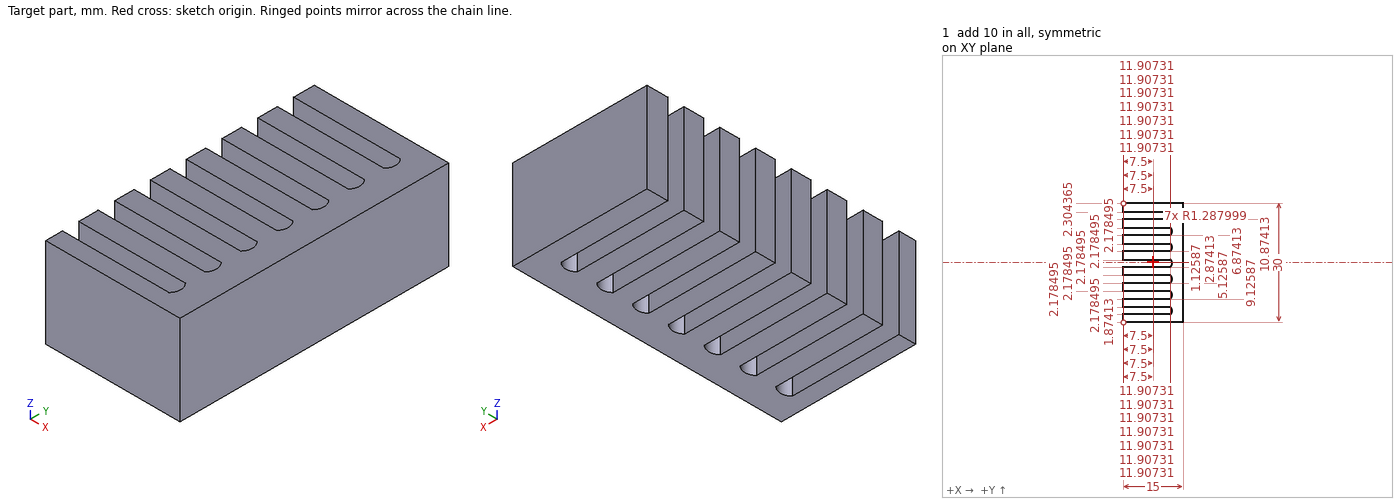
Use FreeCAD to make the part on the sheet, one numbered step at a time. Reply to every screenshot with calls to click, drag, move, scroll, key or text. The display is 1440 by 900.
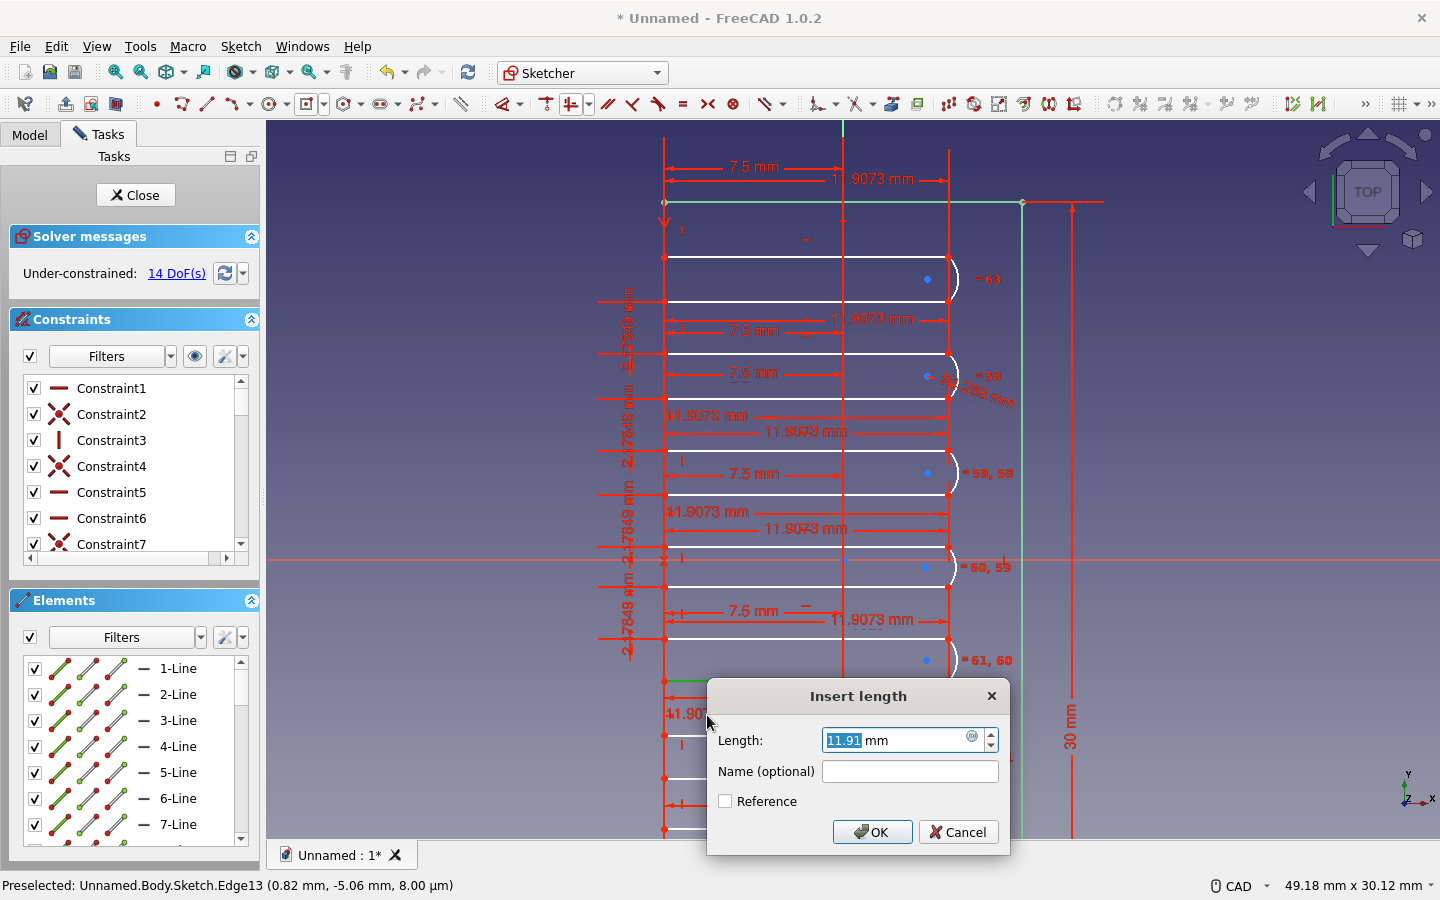
text(11.90731)
key(Return)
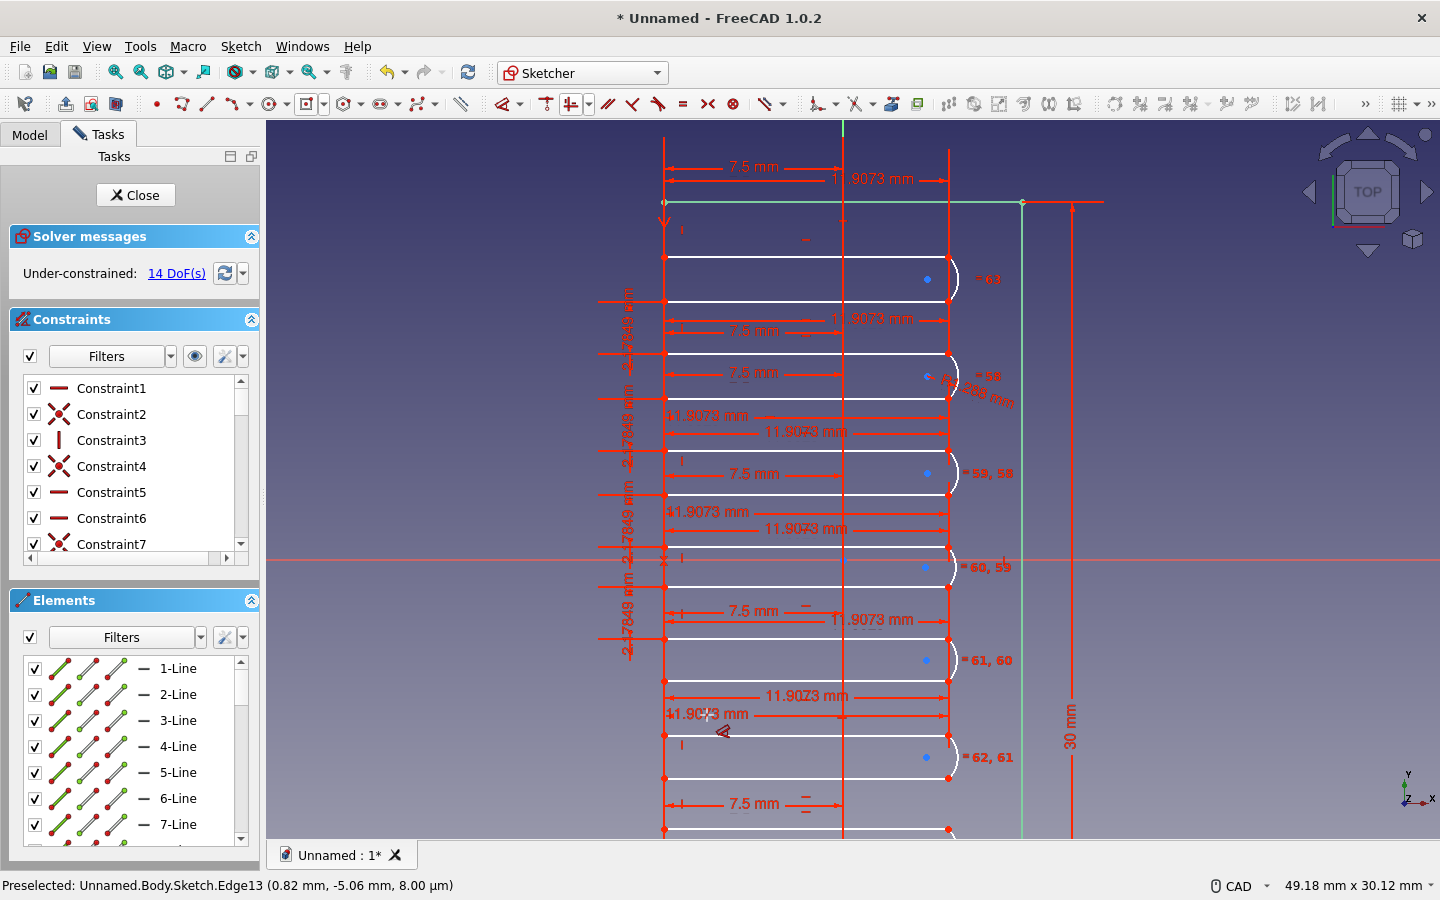
click(664, 698)
click(630, 709)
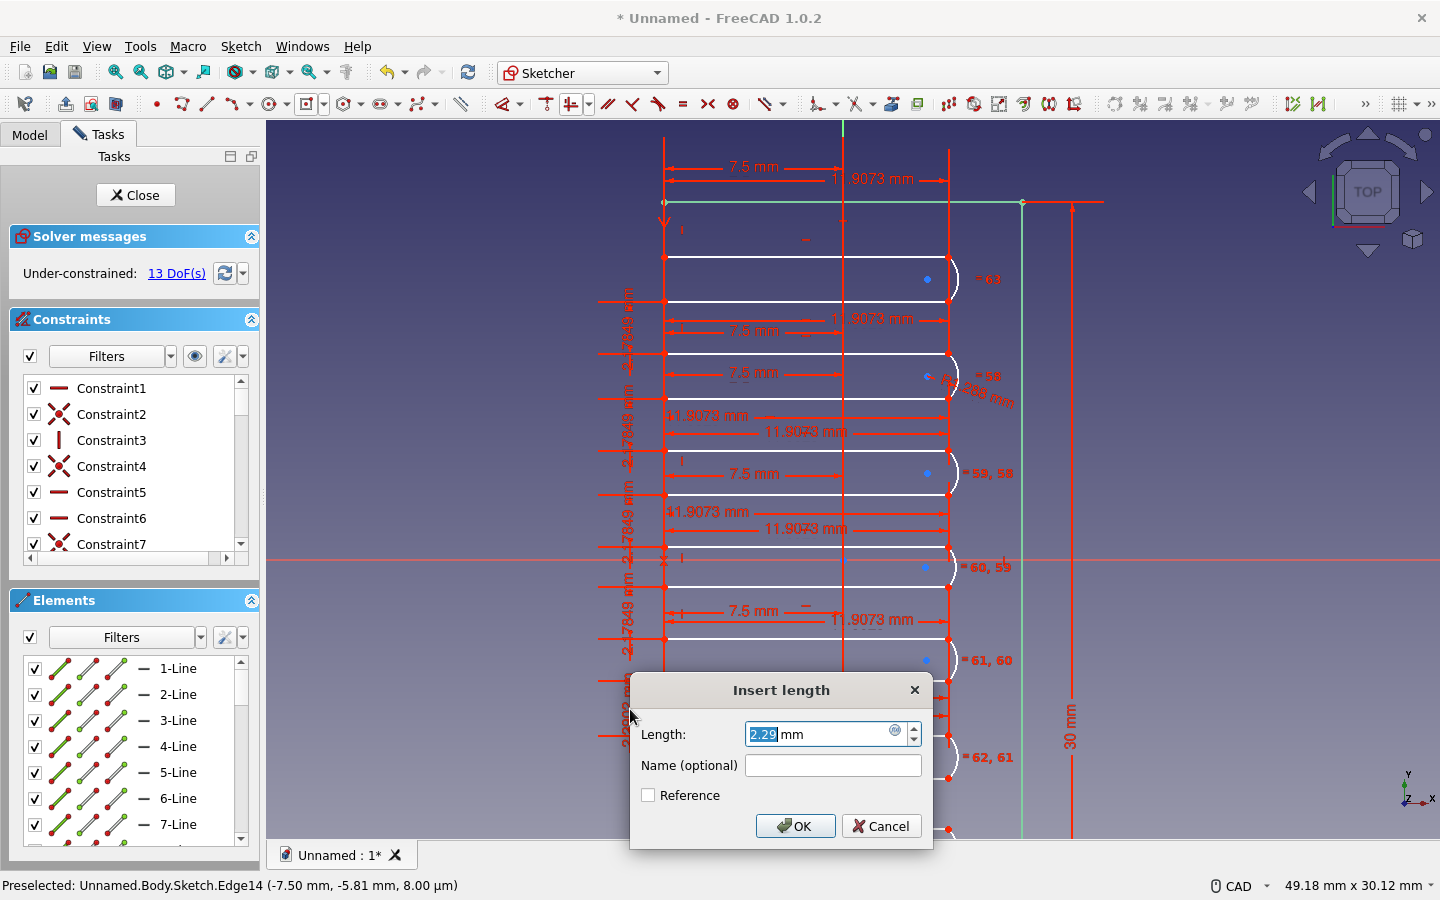
text(2.178495)
key(Return)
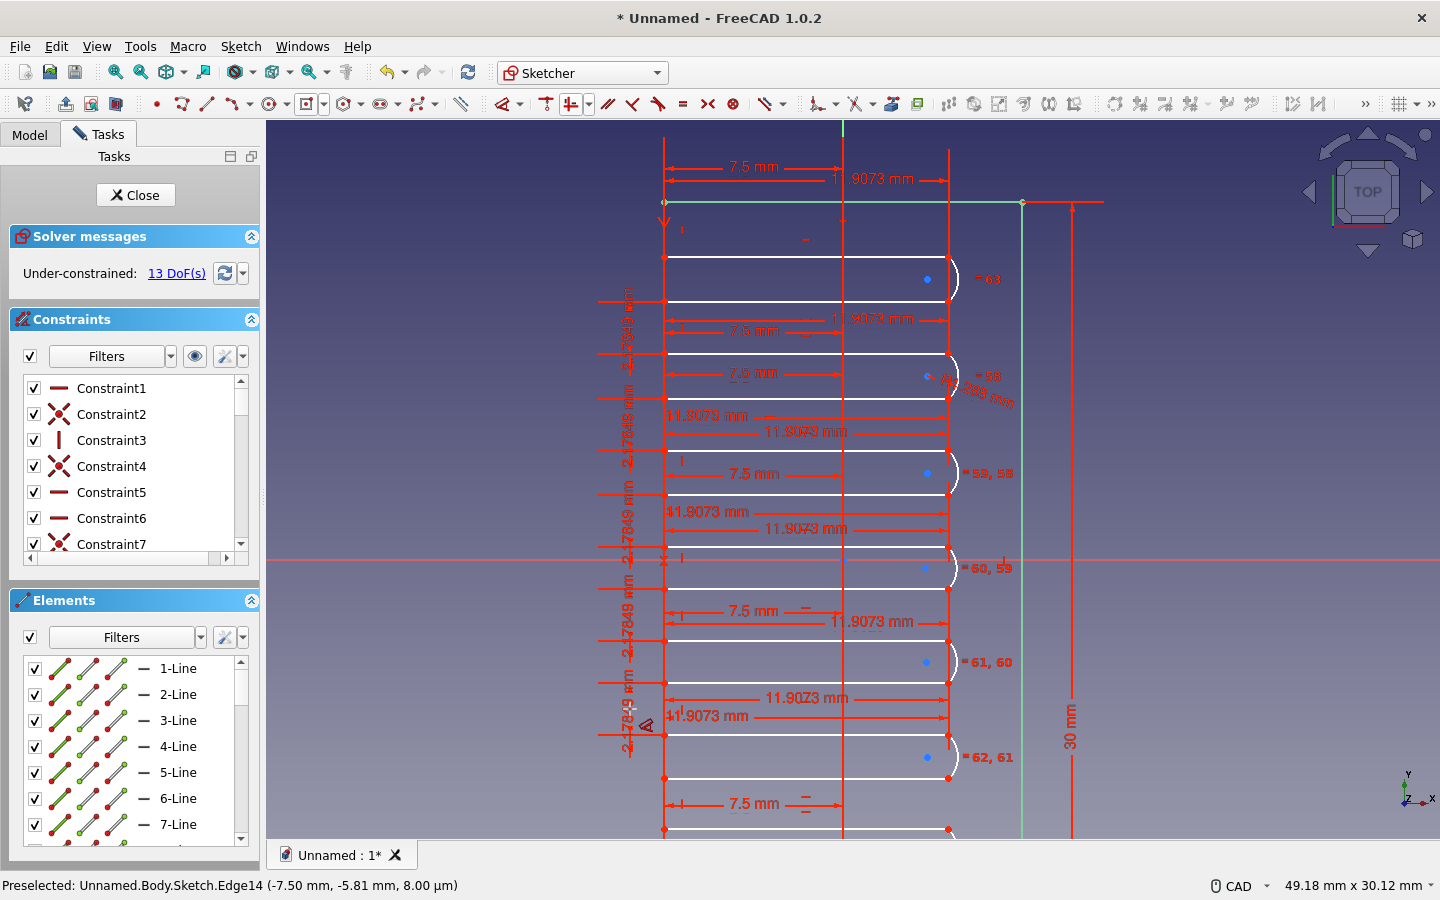
click(750, 735)
click(906, 701)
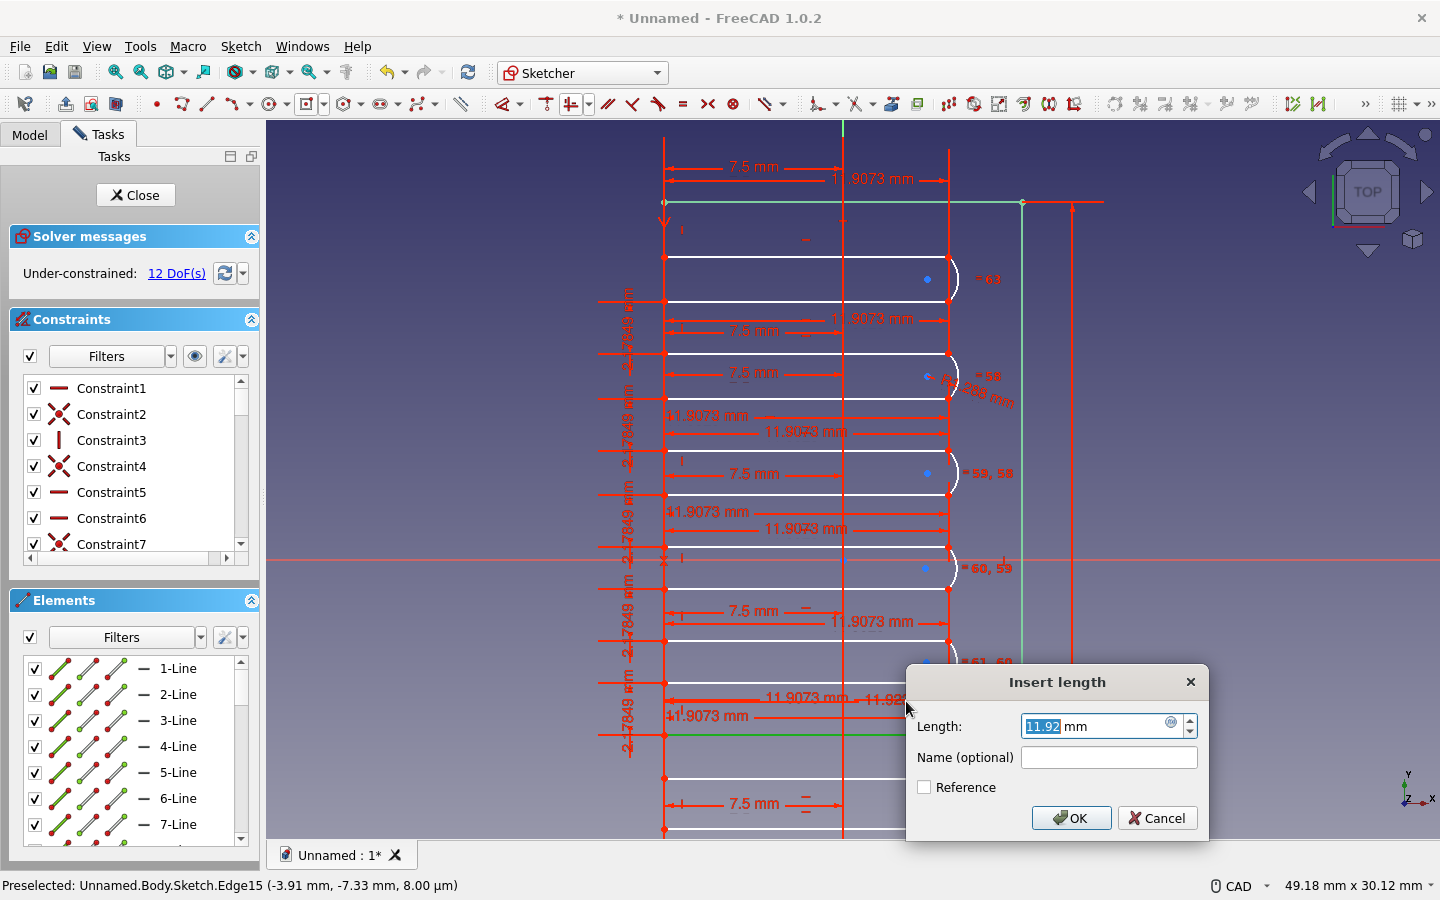
text(11.90731)
key(Return)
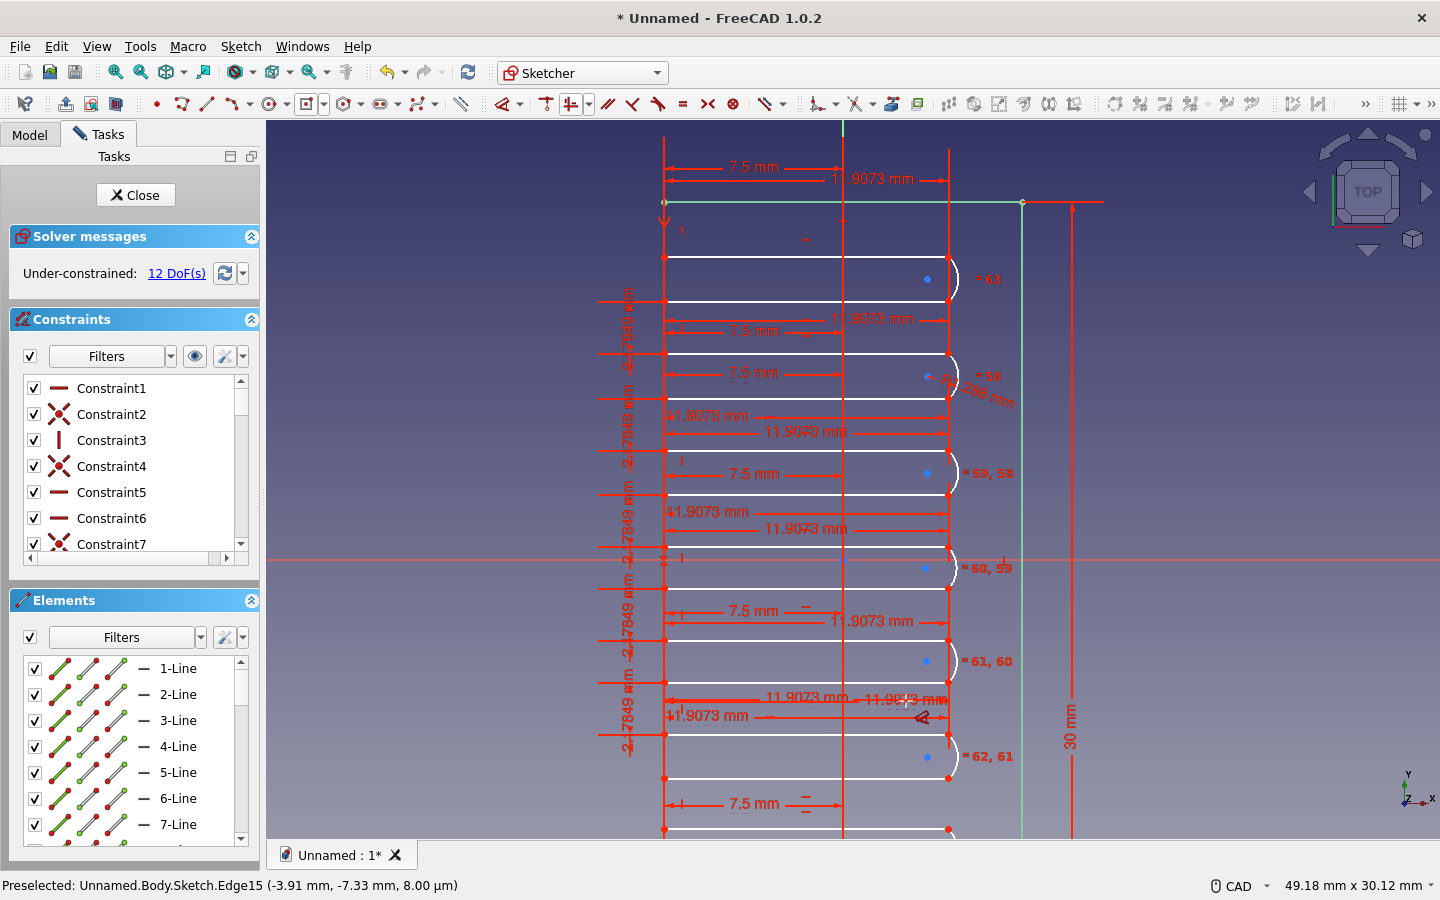
click(864, 779)
click(807, 721)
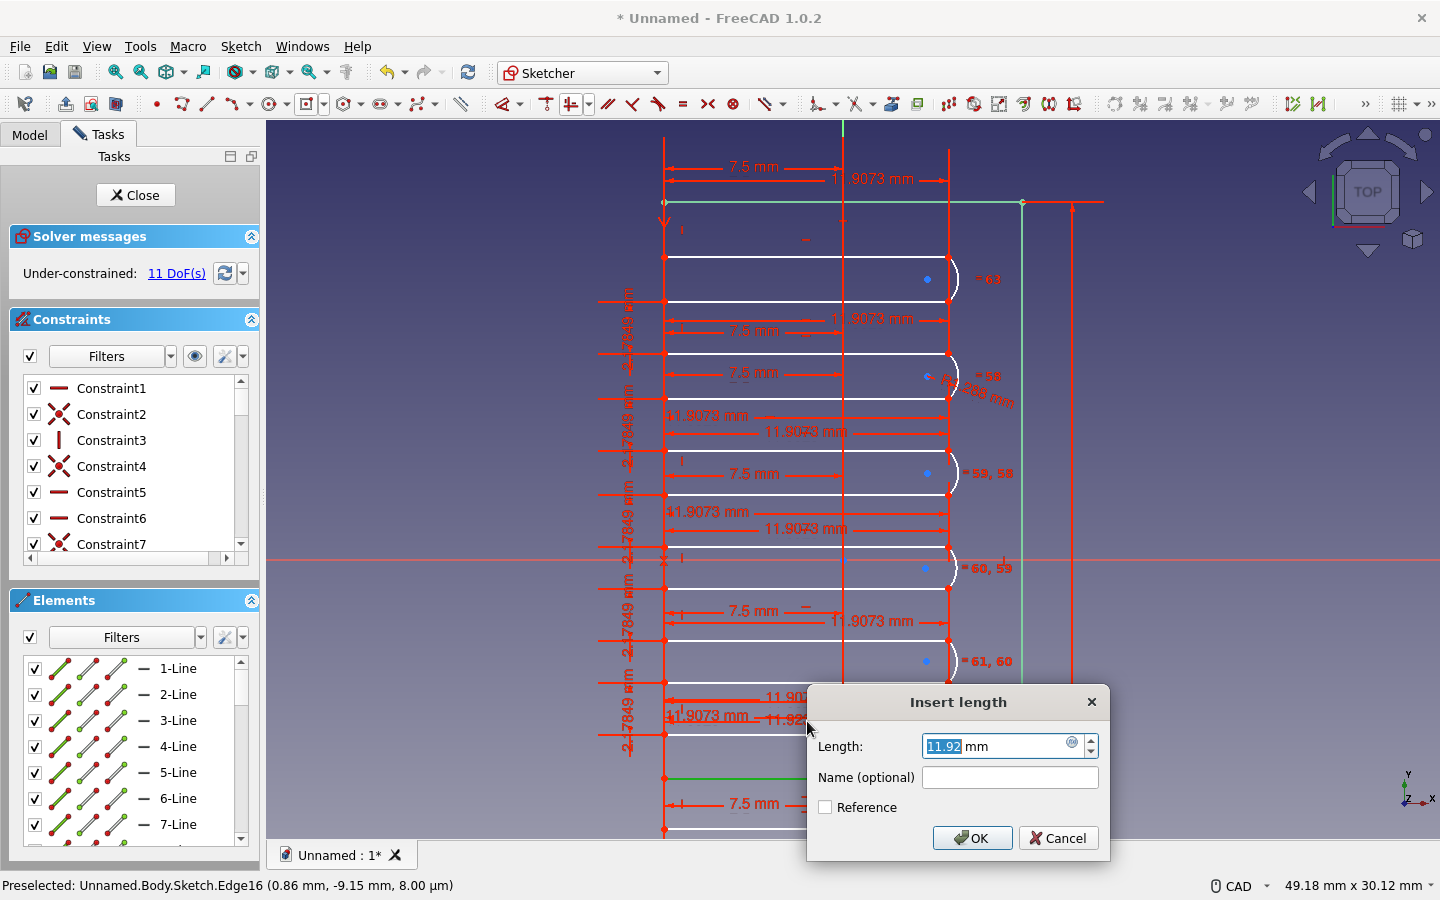
text(11.90731)
key(Return)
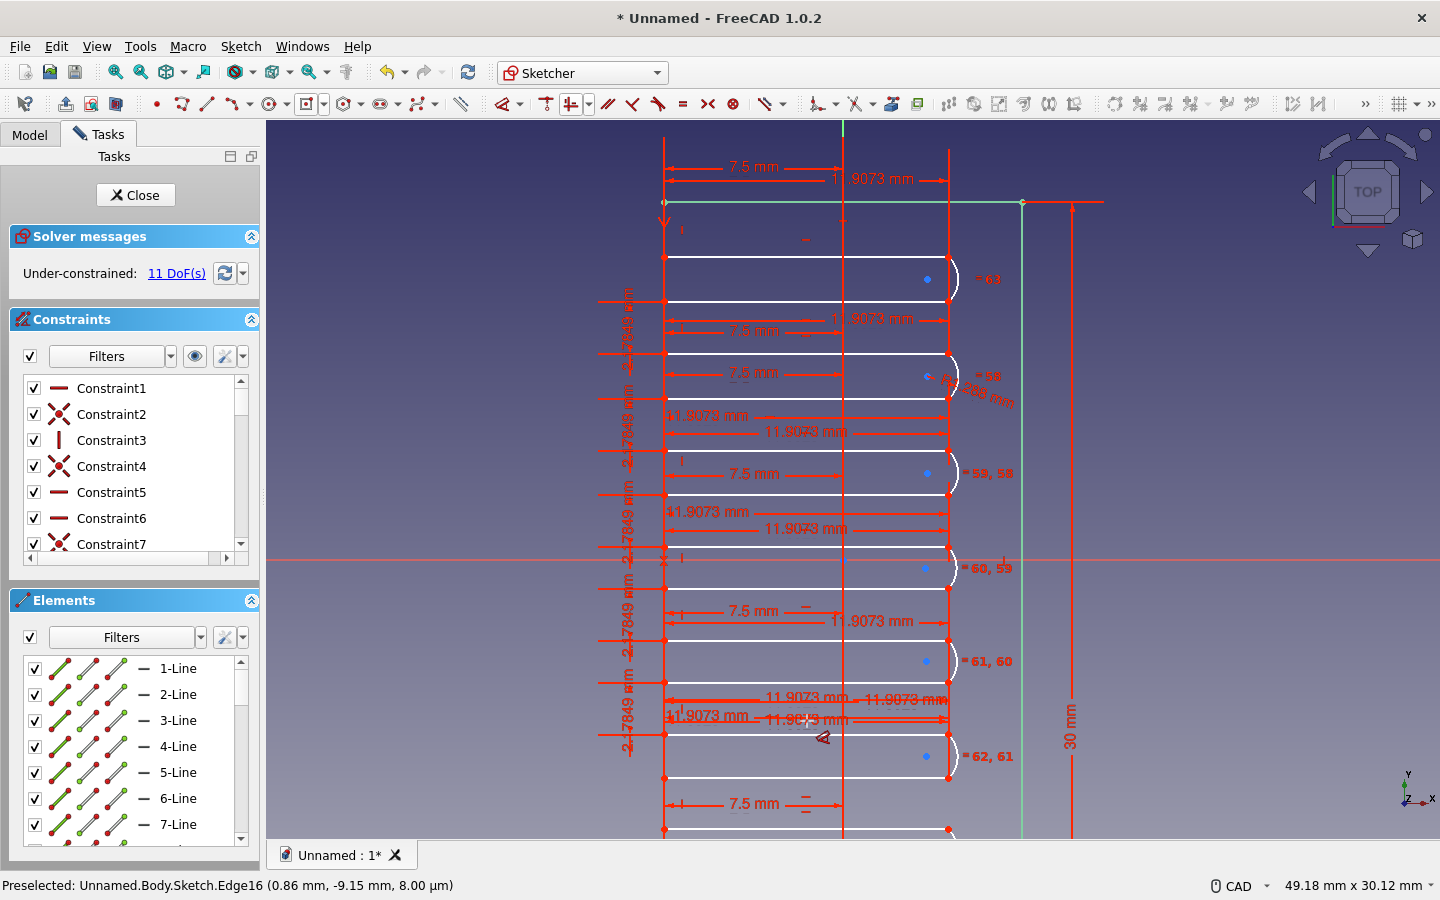
click(664, 794)
click(630, 795)